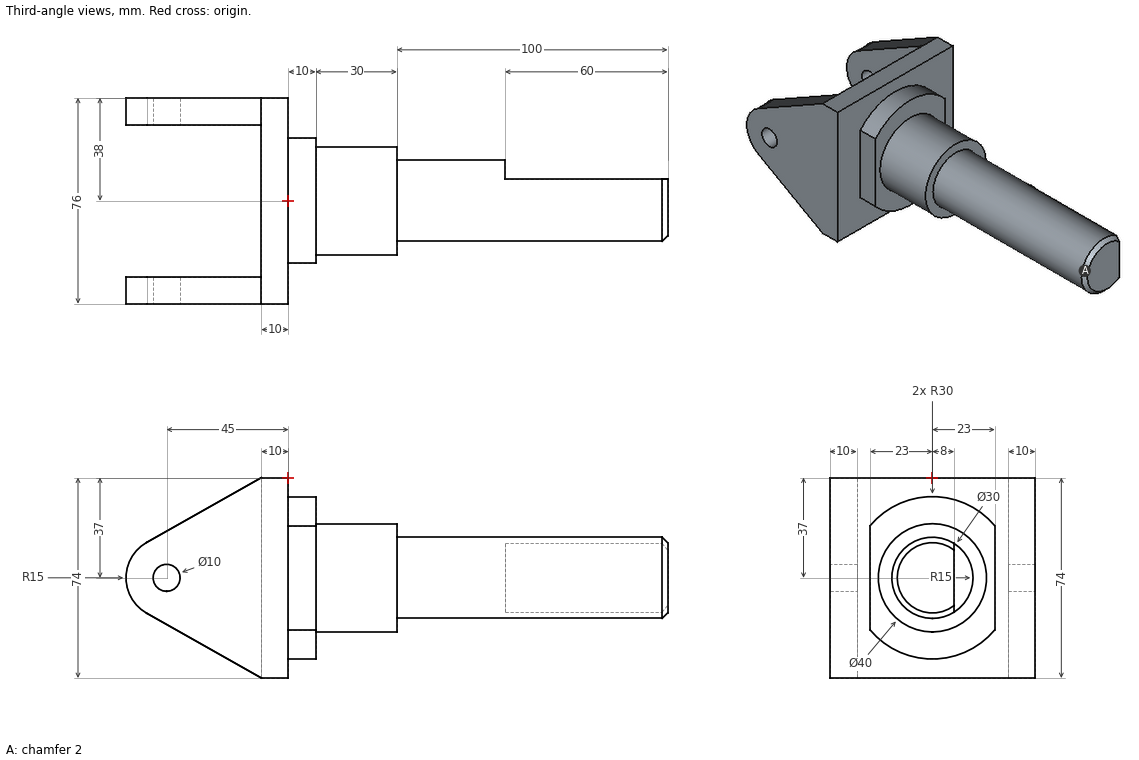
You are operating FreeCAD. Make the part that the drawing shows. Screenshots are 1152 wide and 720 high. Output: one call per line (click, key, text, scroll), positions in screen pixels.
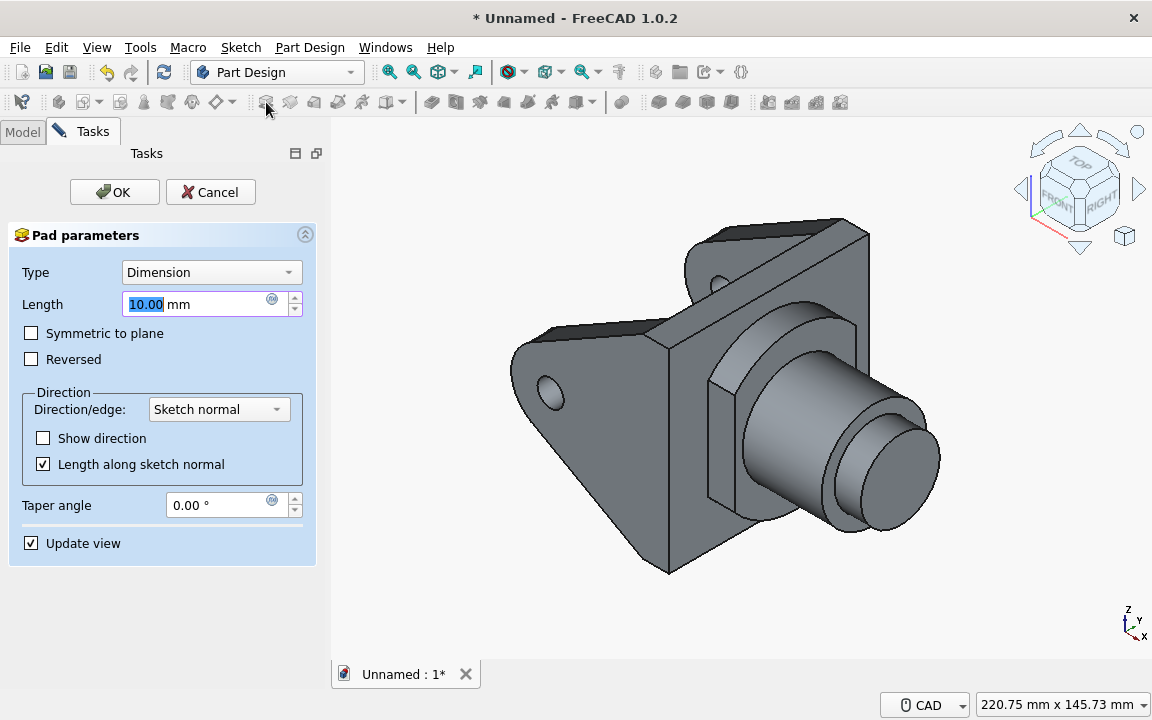
text(100)
key(Tab)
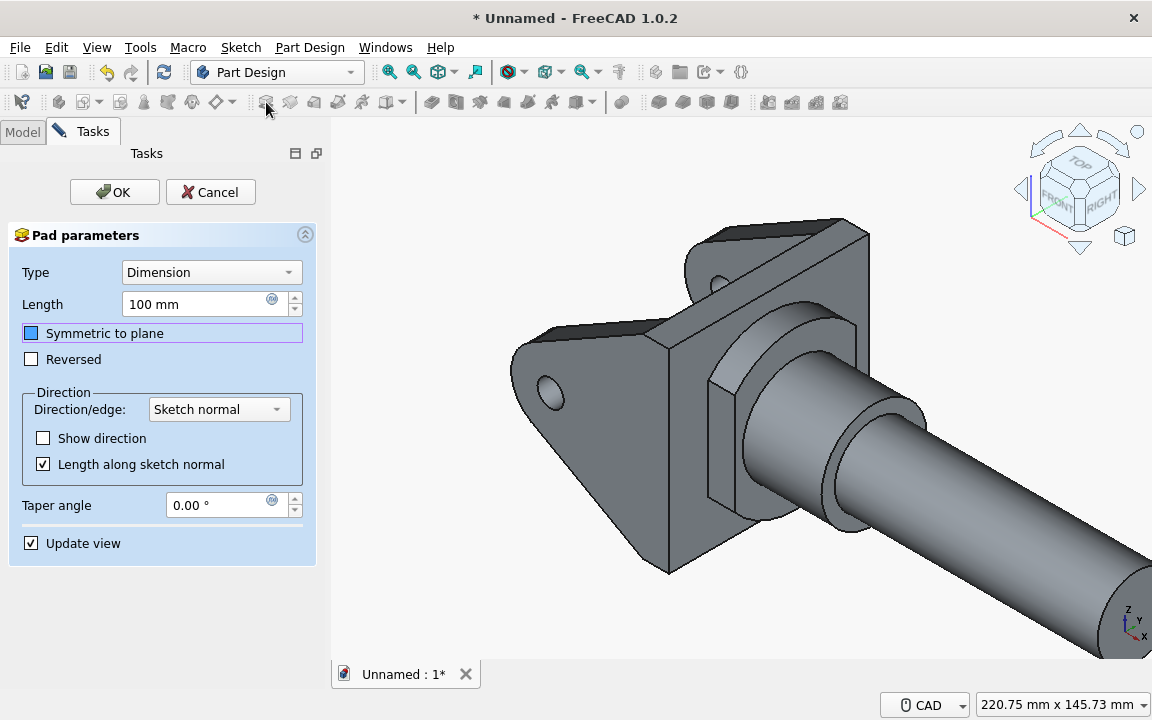
click(115, 192)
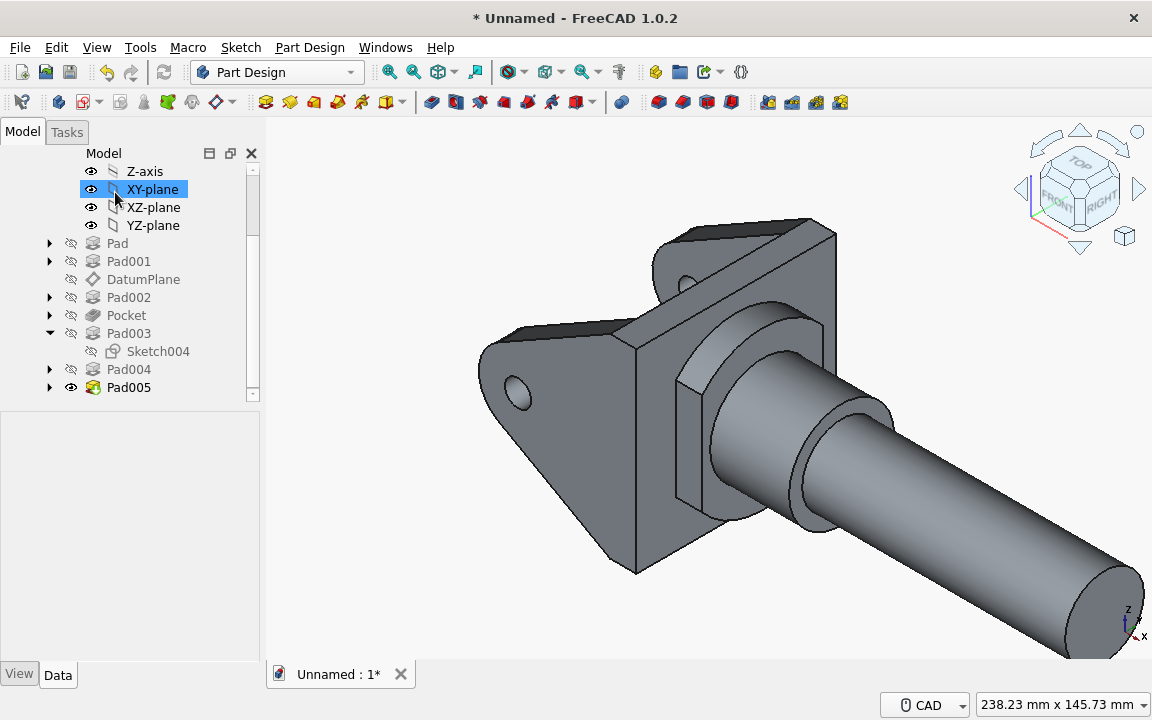
click(390, 72)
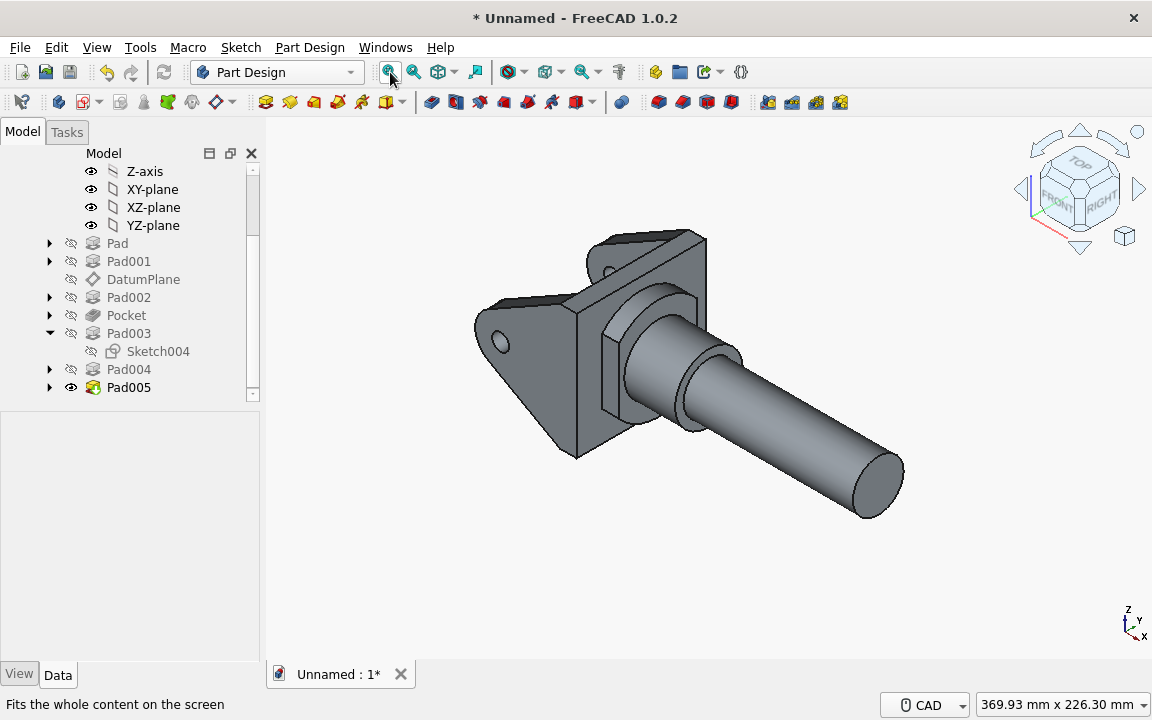
scroll(160, 275, down, 3)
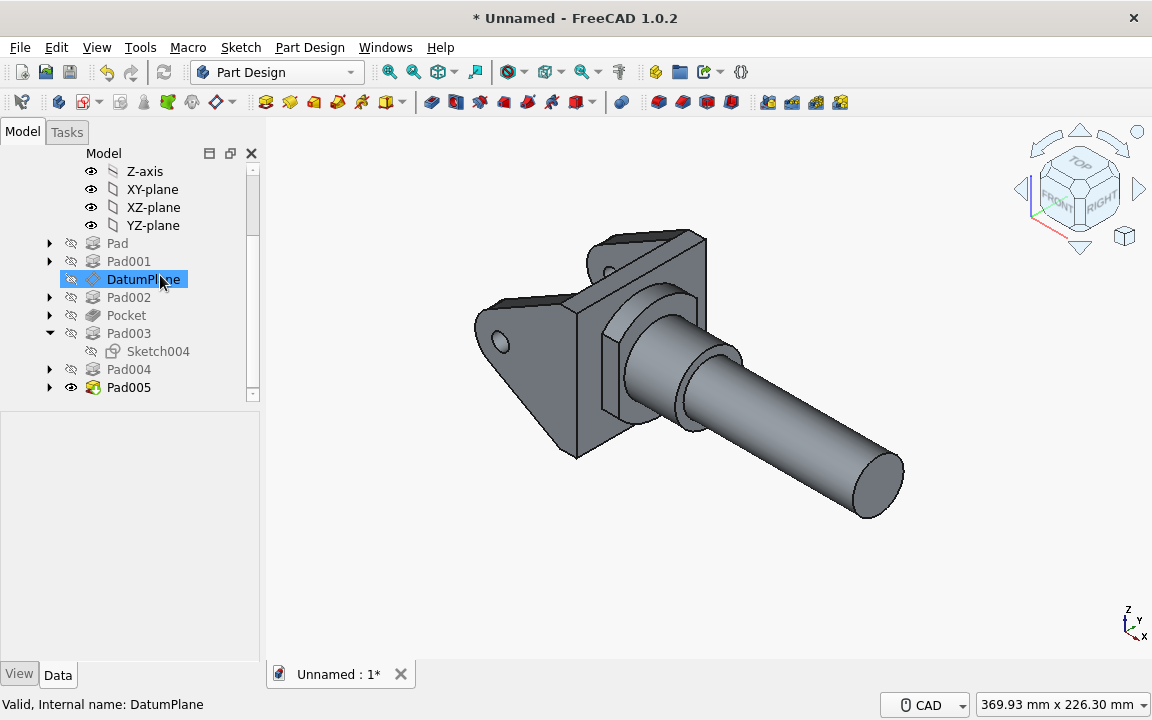
scroll(160, 275, up, 15)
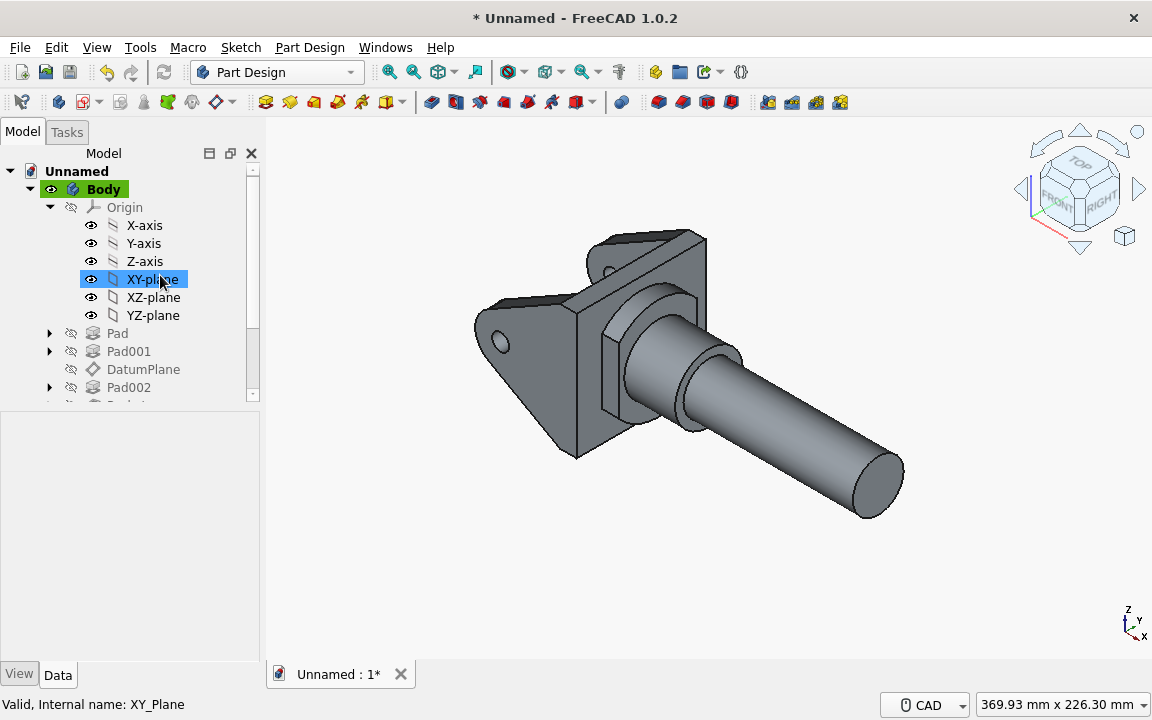
click(136, 315)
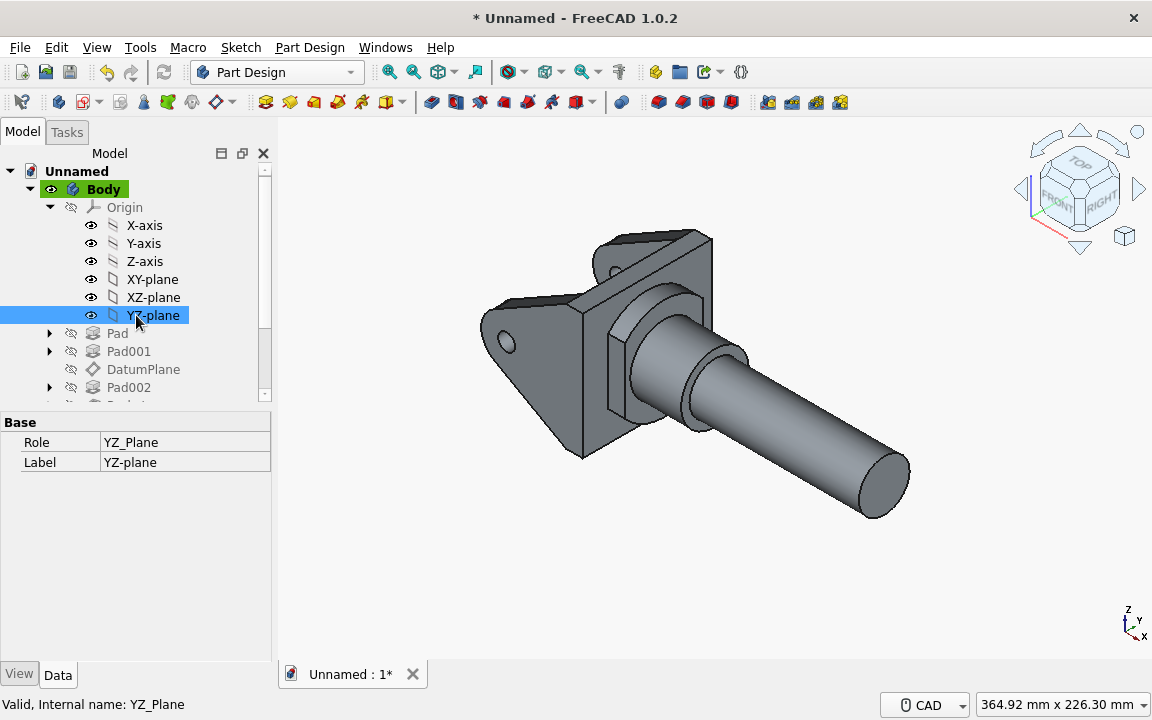
click(216, 102)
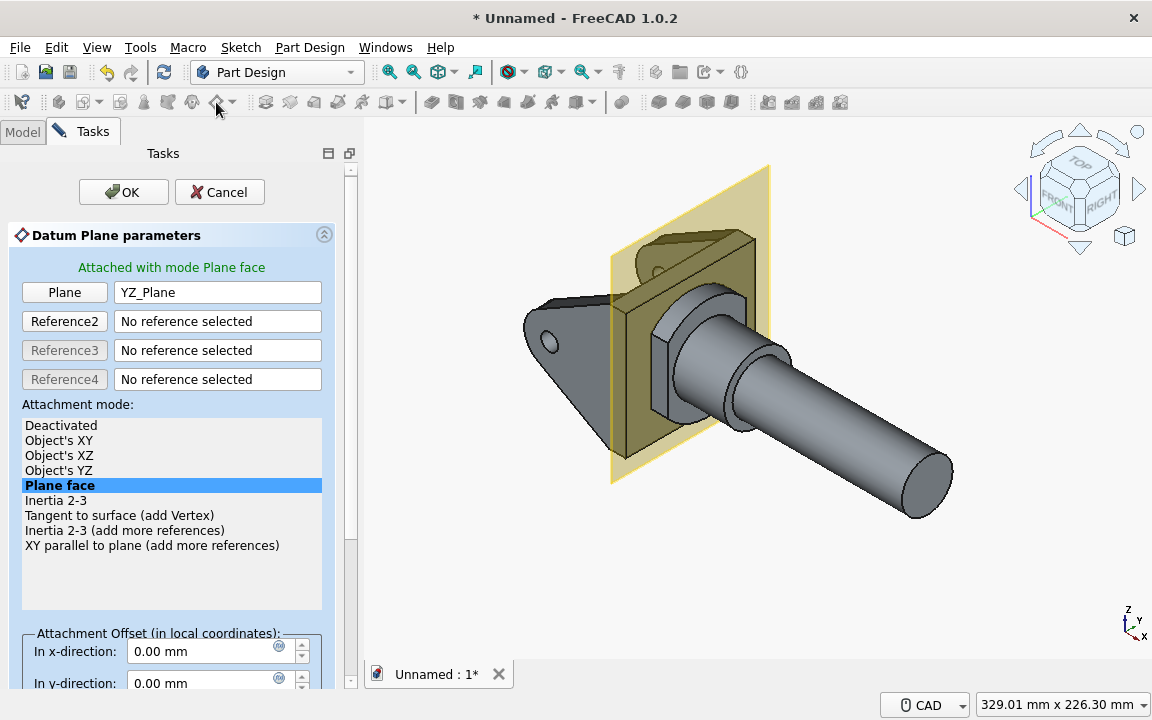
scroll(351, 426, down, 2)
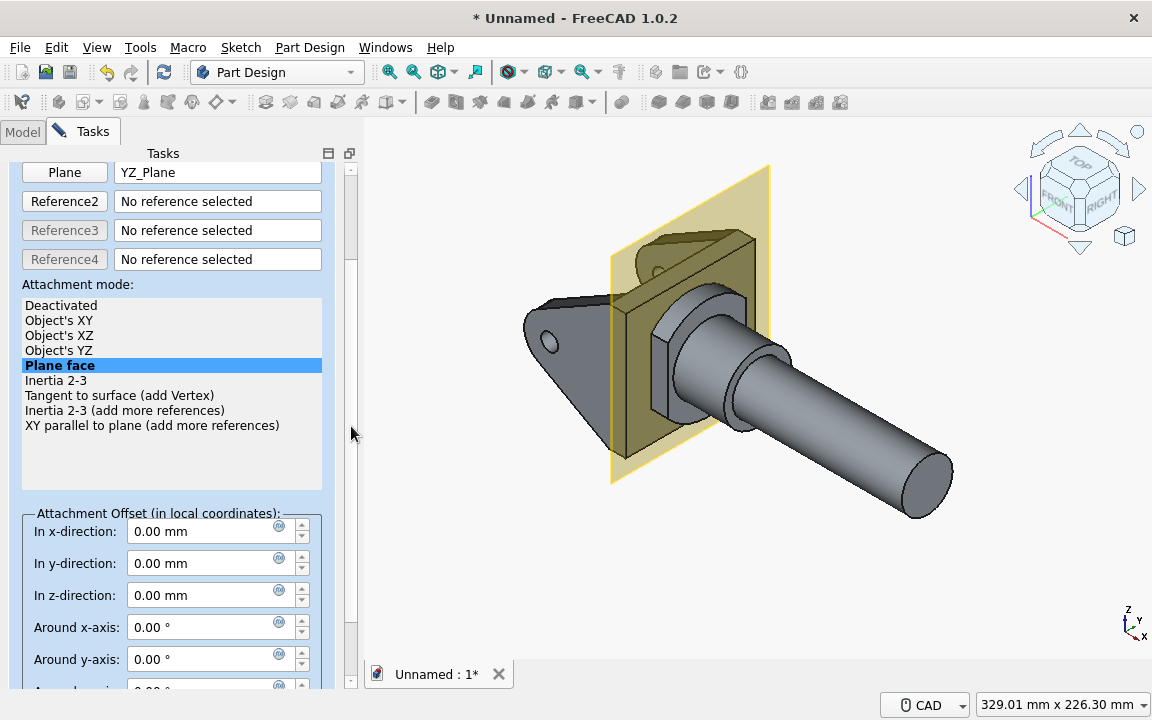
triple_click(210, 595)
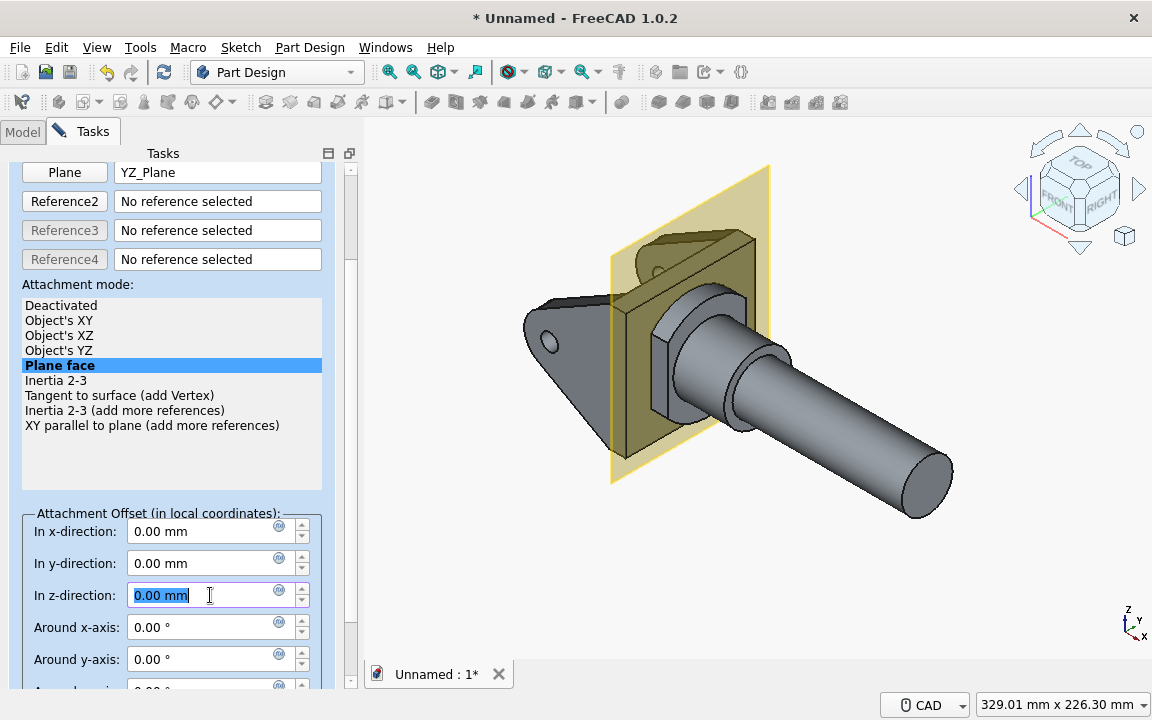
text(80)
key(Tab)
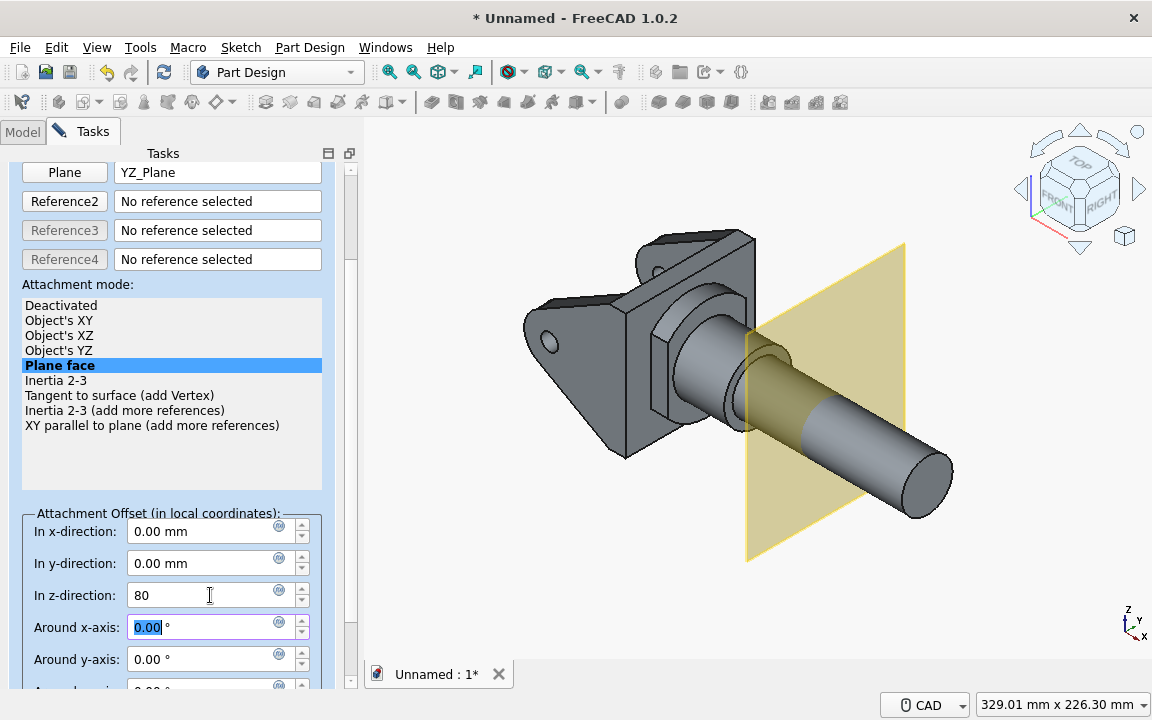
scroll(351, 426, up, 3)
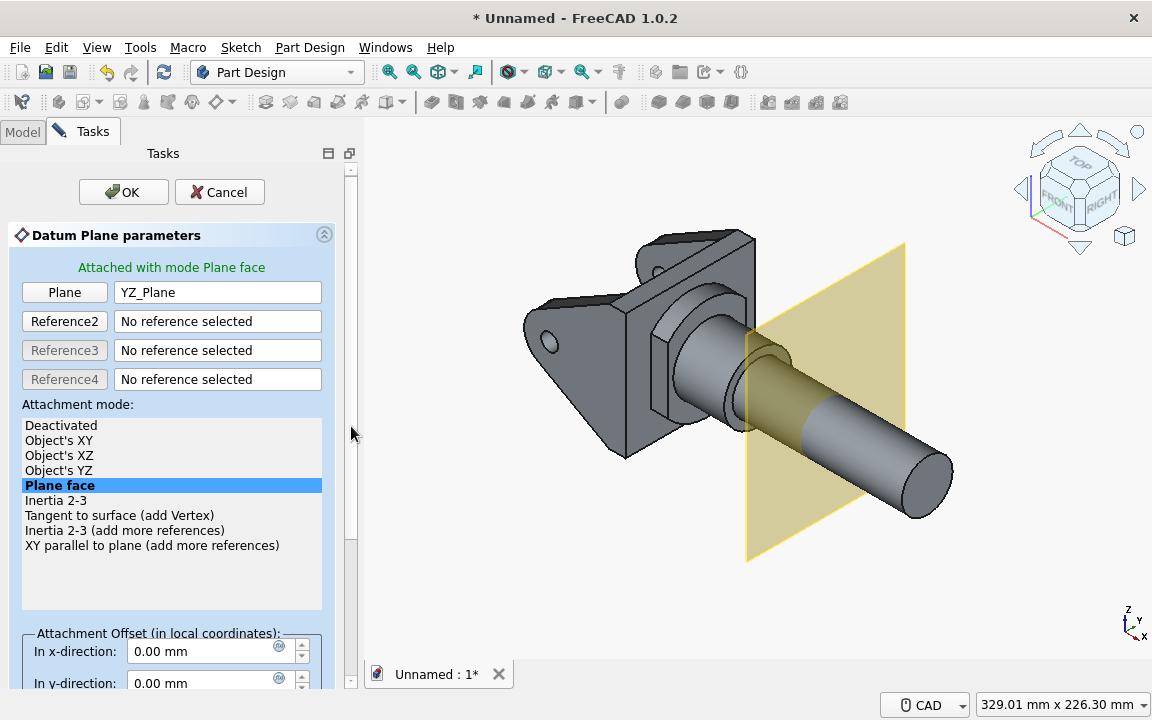
click(124, 192)